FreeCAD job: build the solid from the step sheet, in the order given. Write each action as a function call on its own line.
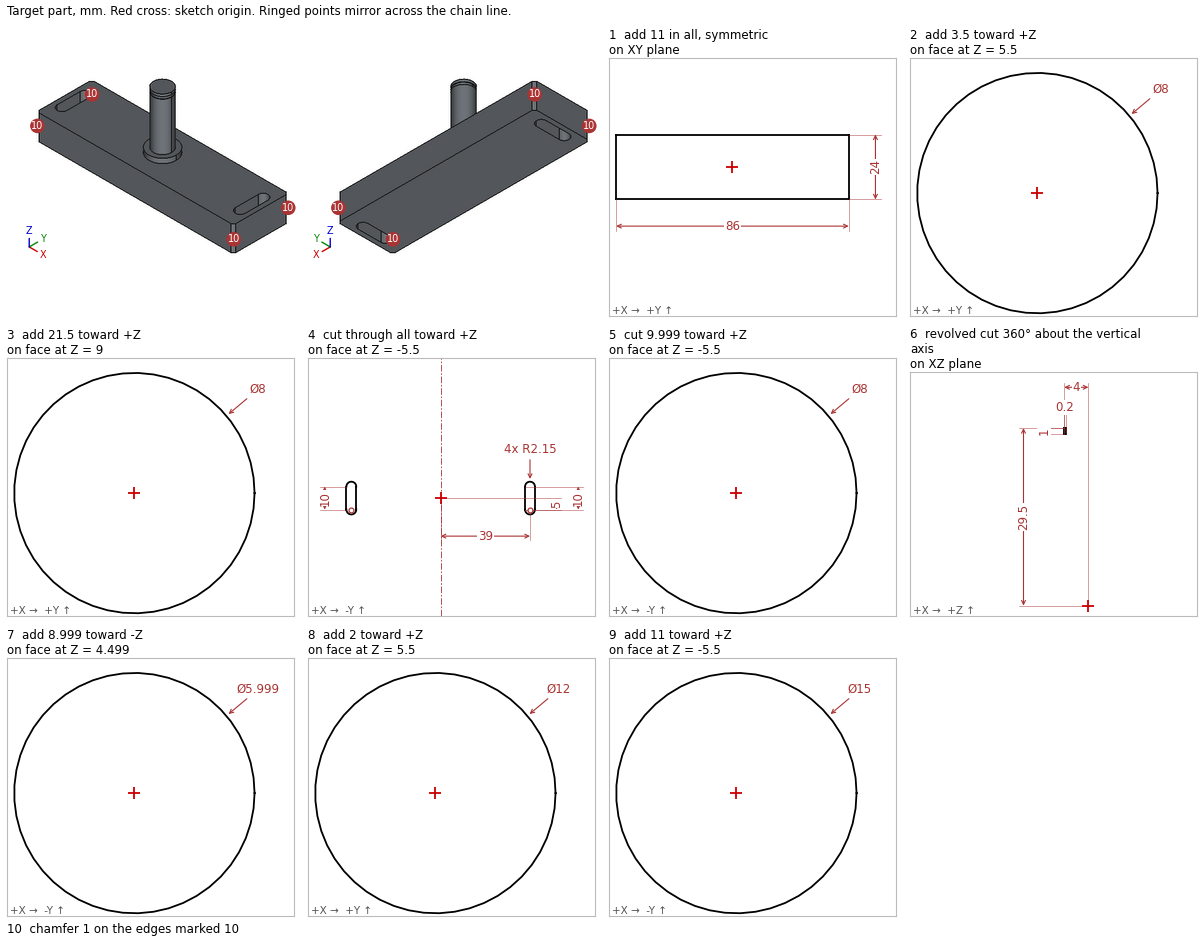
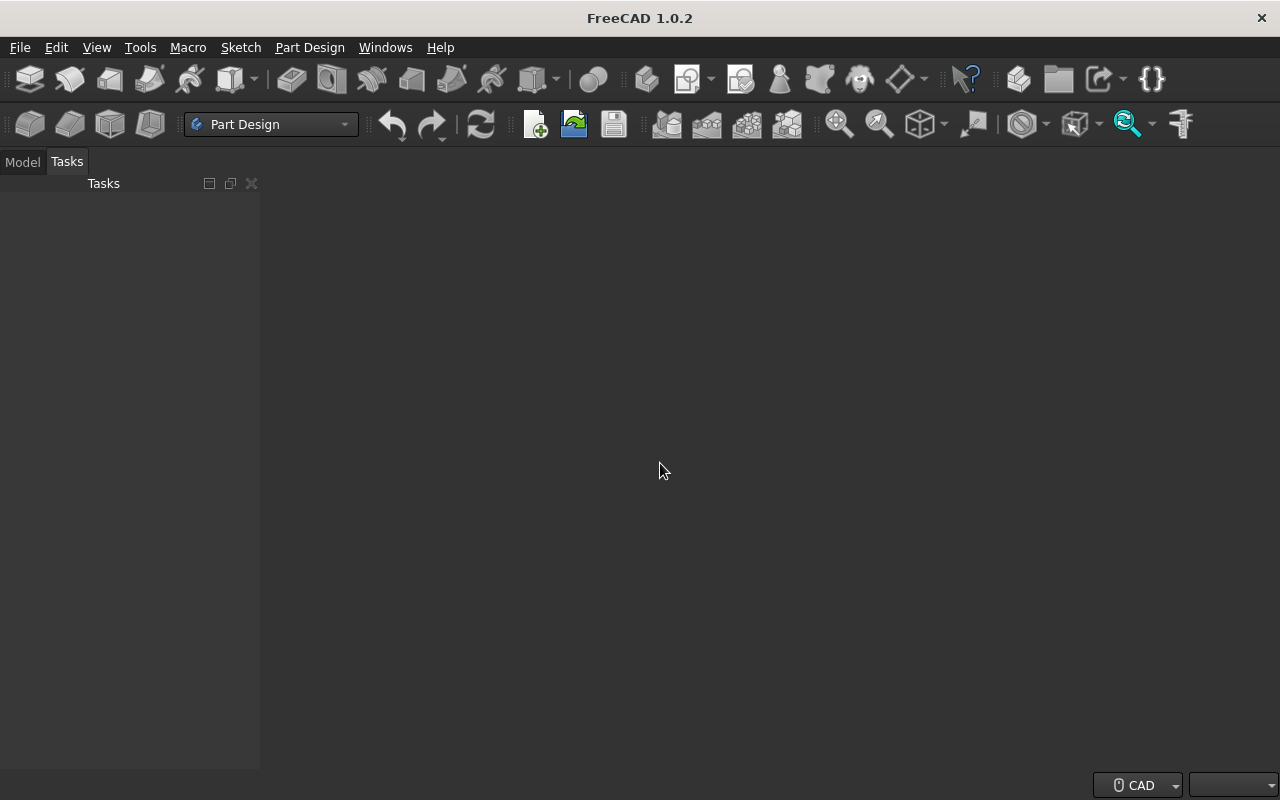
click(534, 124)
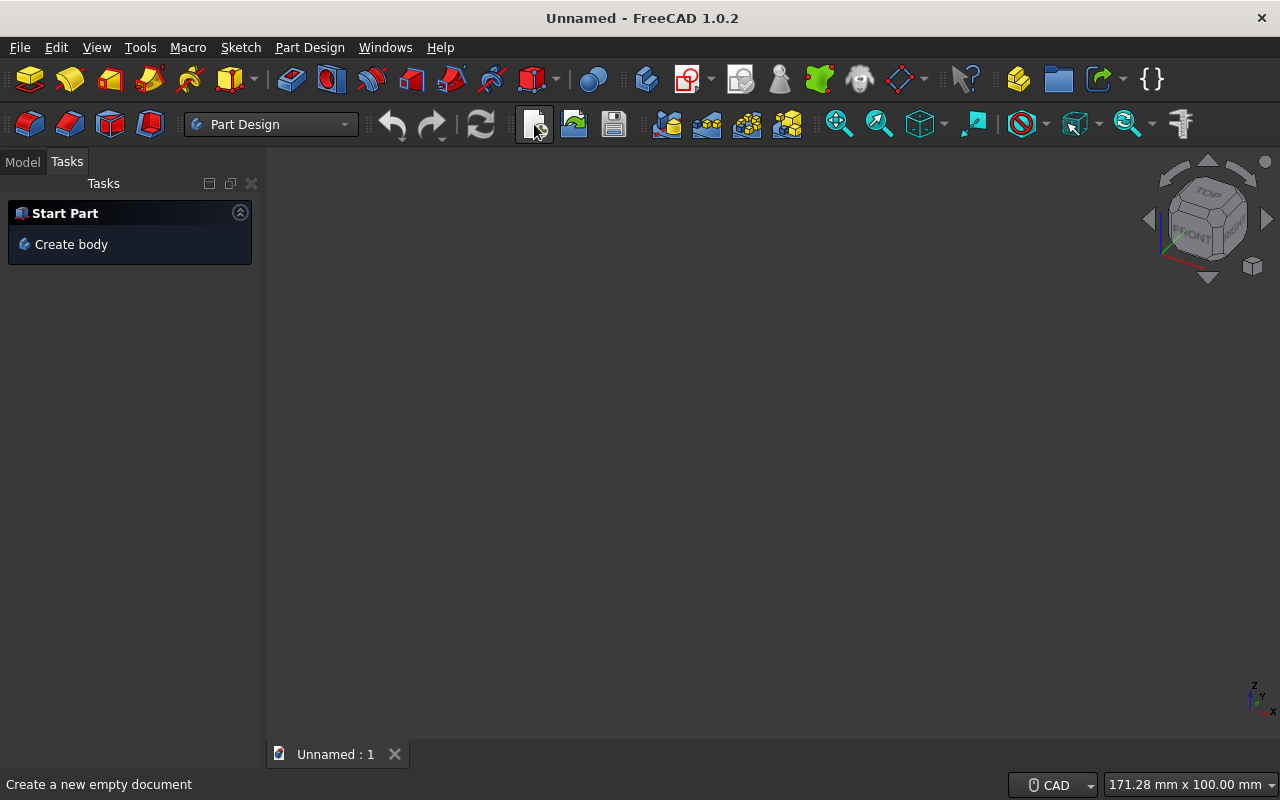
click(688, 80)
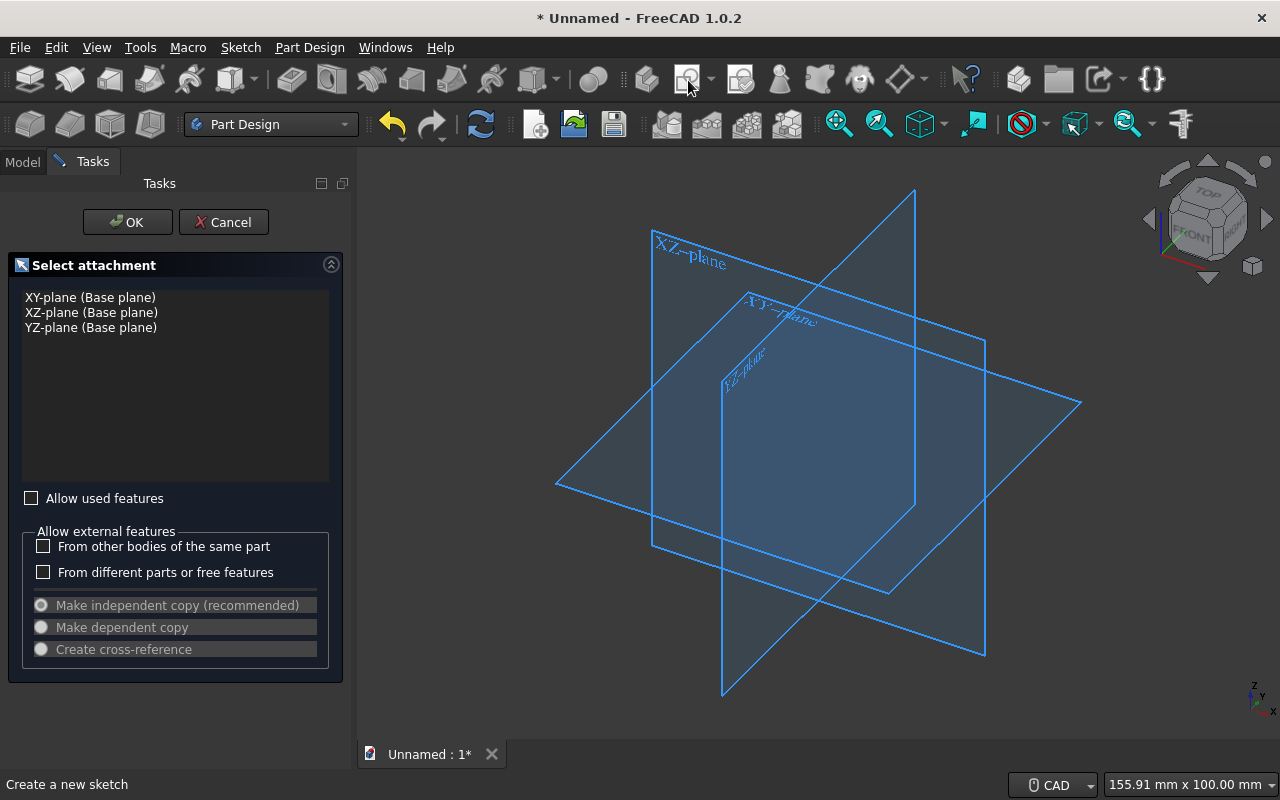
click(82, 298)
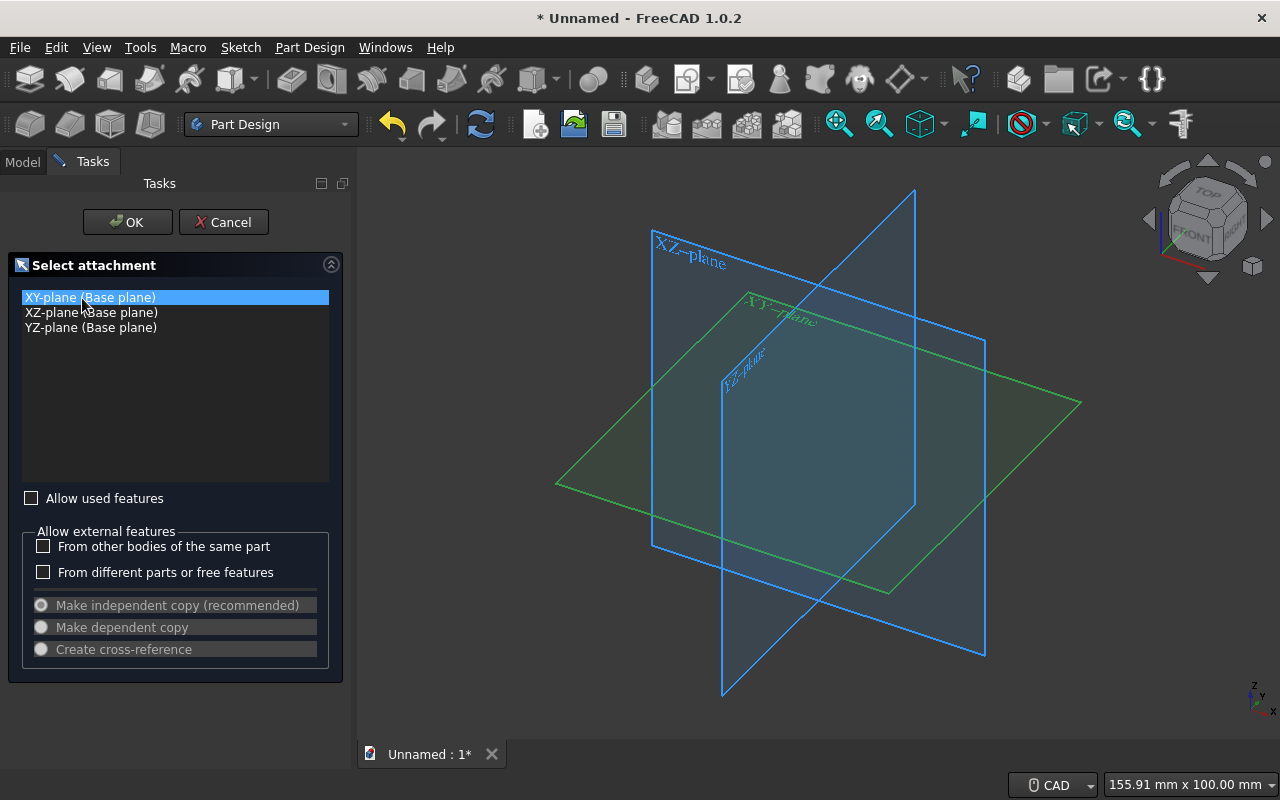
click(128, 222)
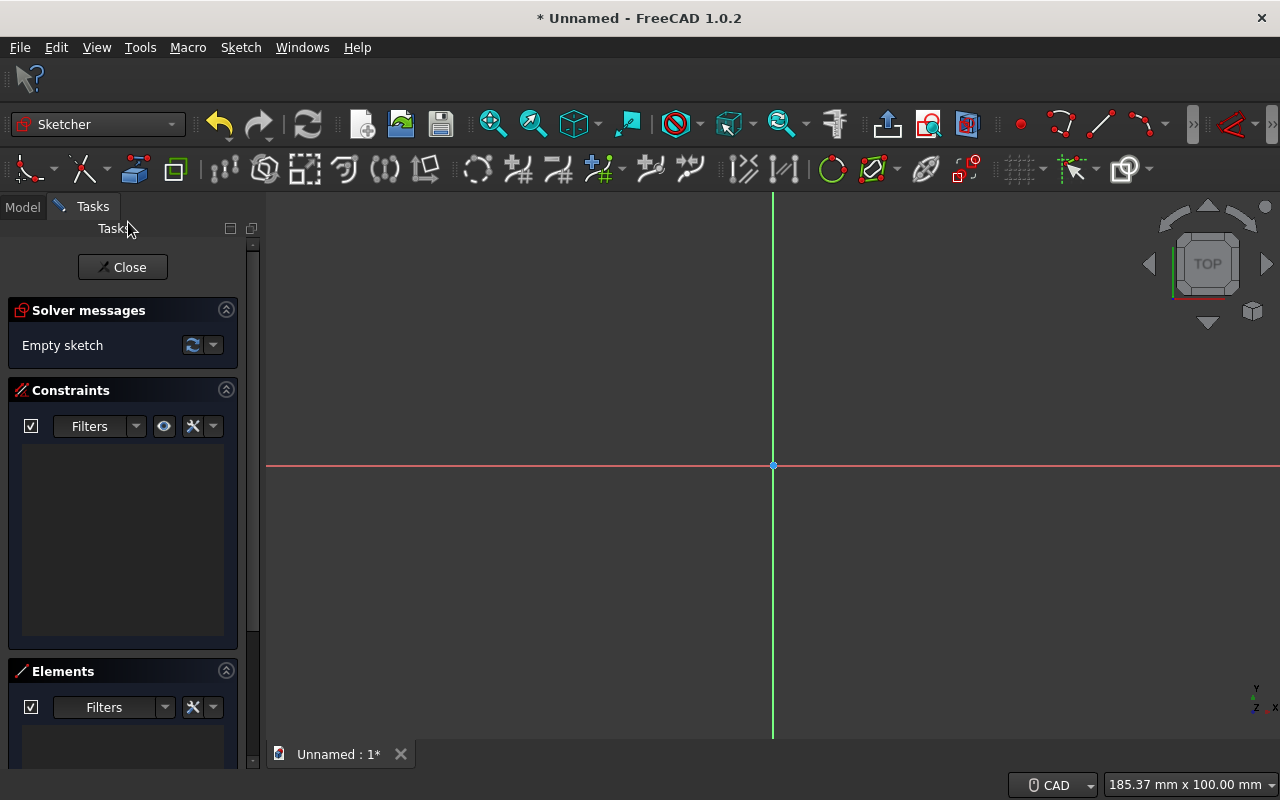
key(g)
key(v)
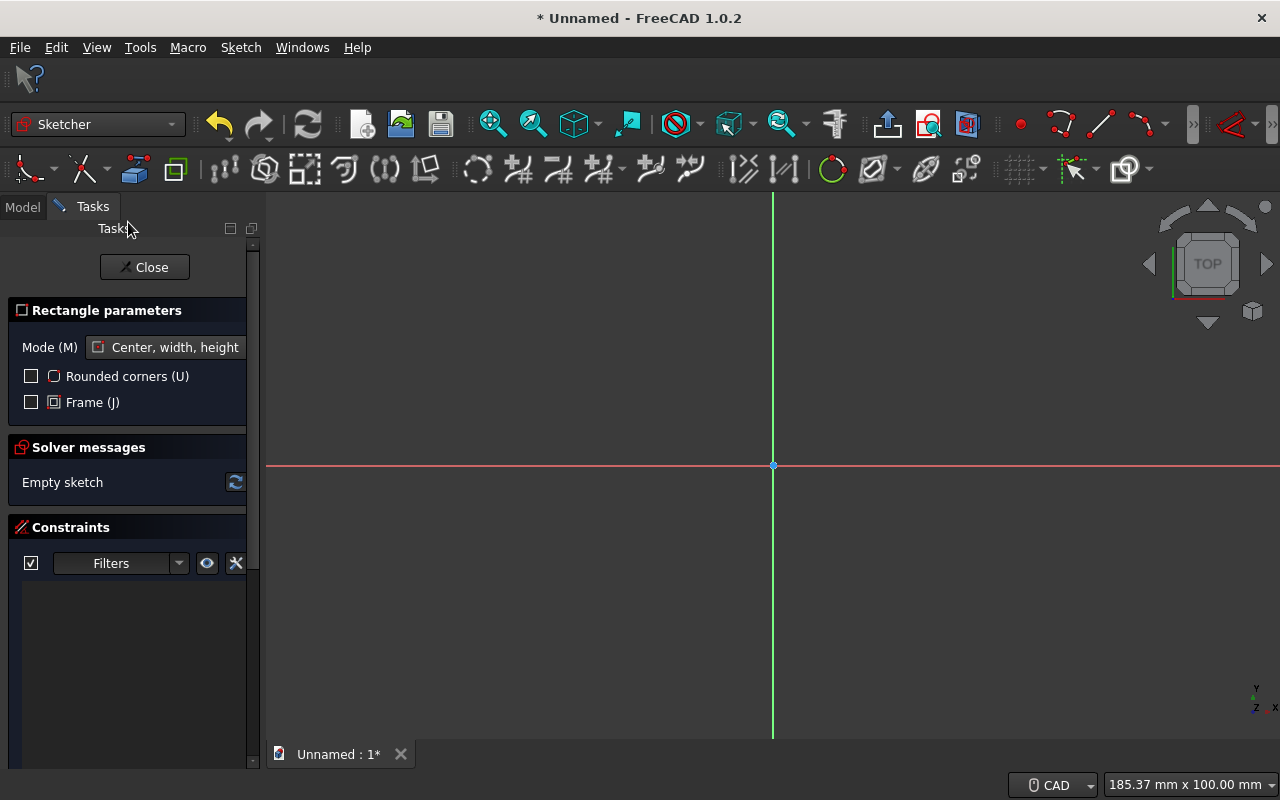
click(773, 466)
move(1008, 400)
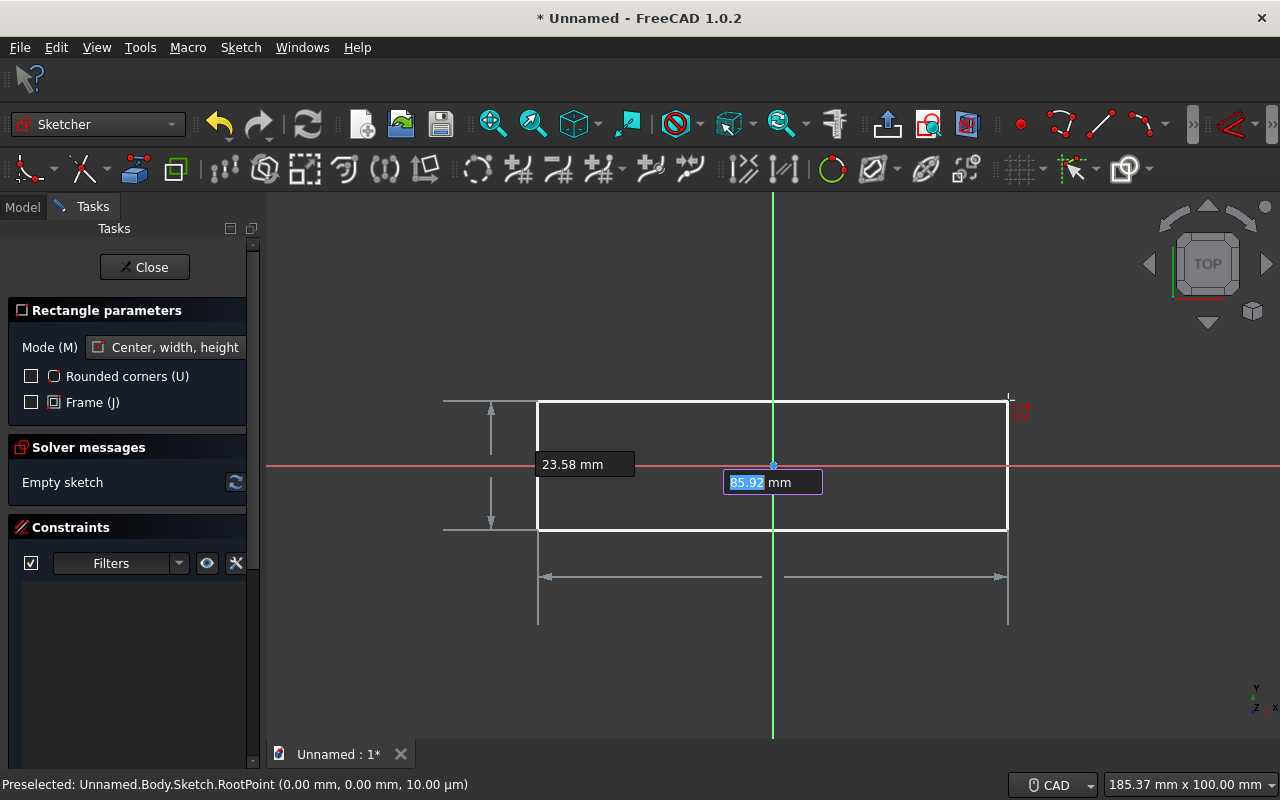
text(86)
key(Tab)
text(24)
key(Return)
key(Escape)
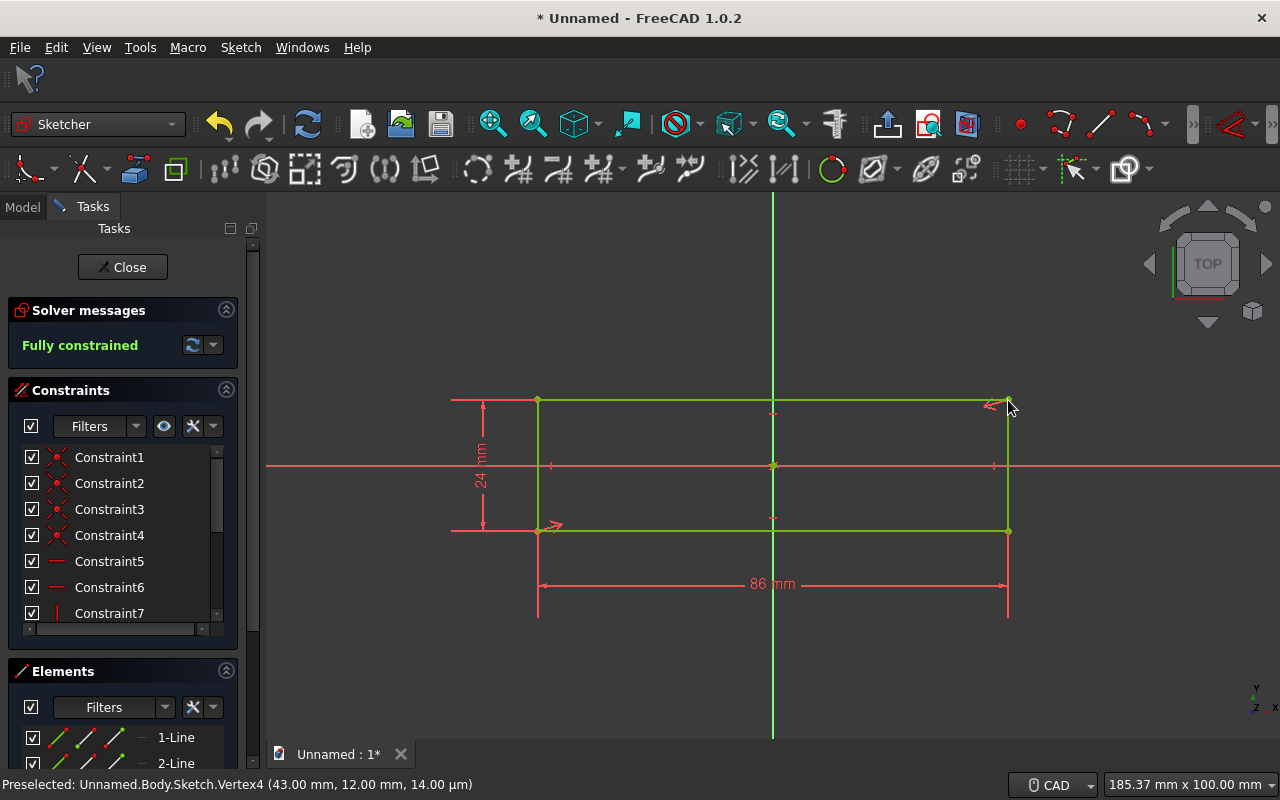
click(123, 267)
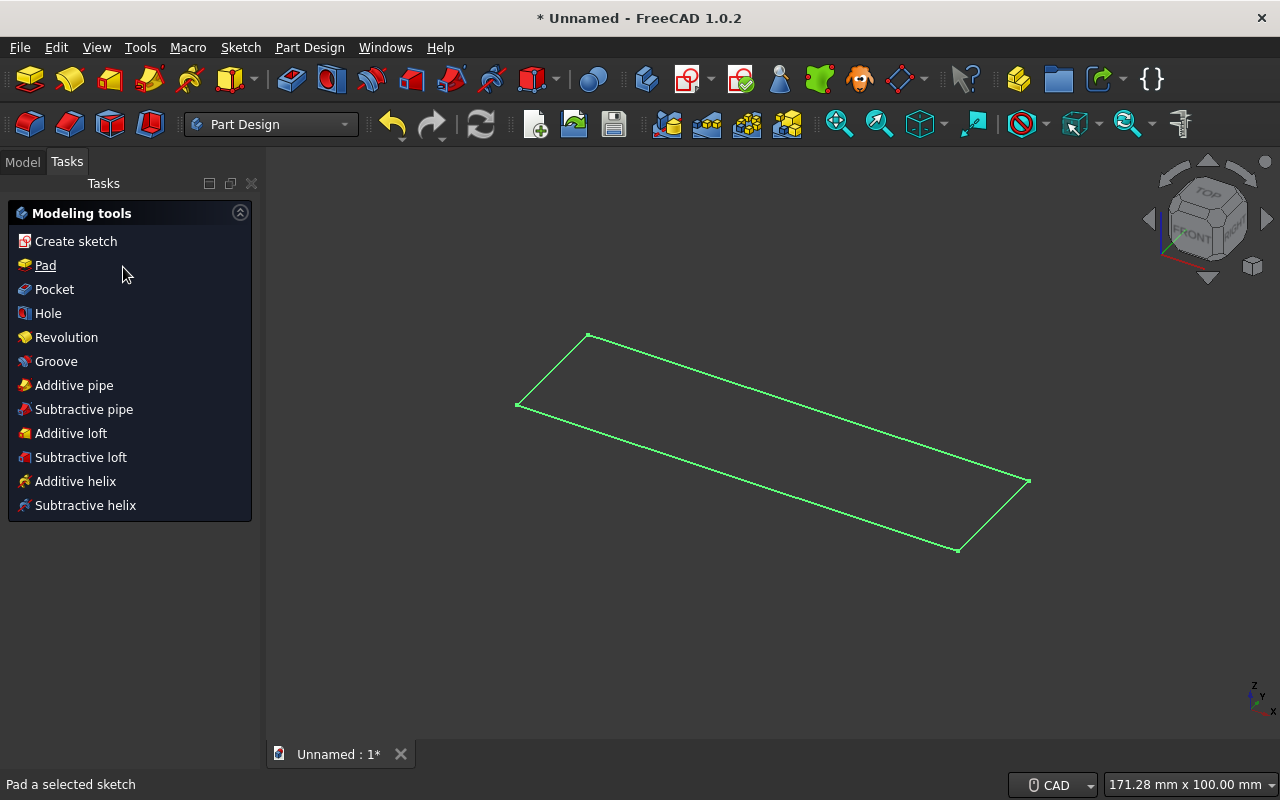
click(30, 80)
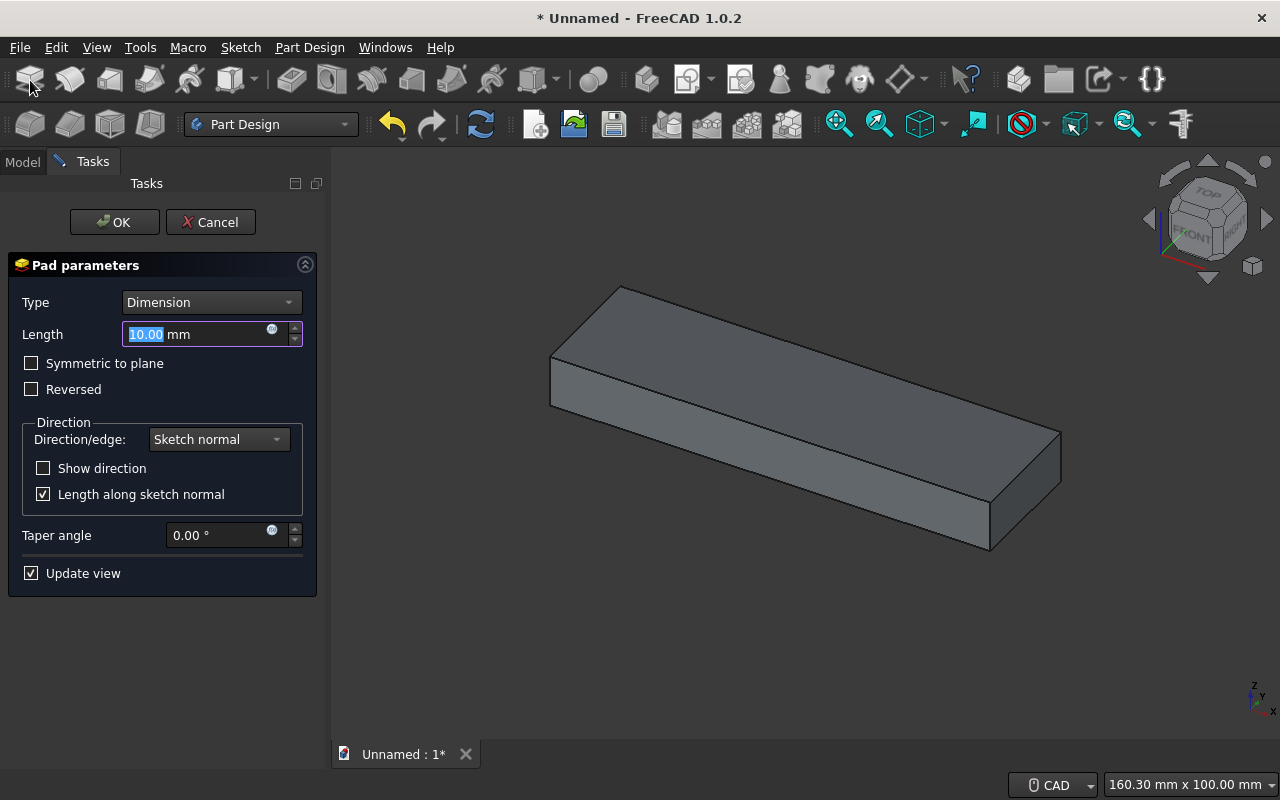
text(11)
key(Tab)